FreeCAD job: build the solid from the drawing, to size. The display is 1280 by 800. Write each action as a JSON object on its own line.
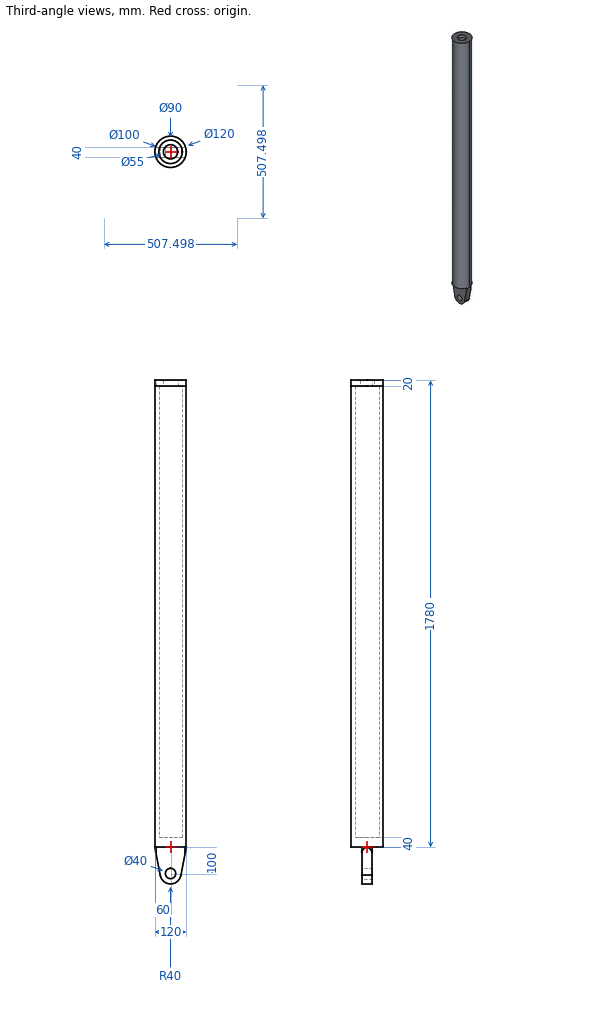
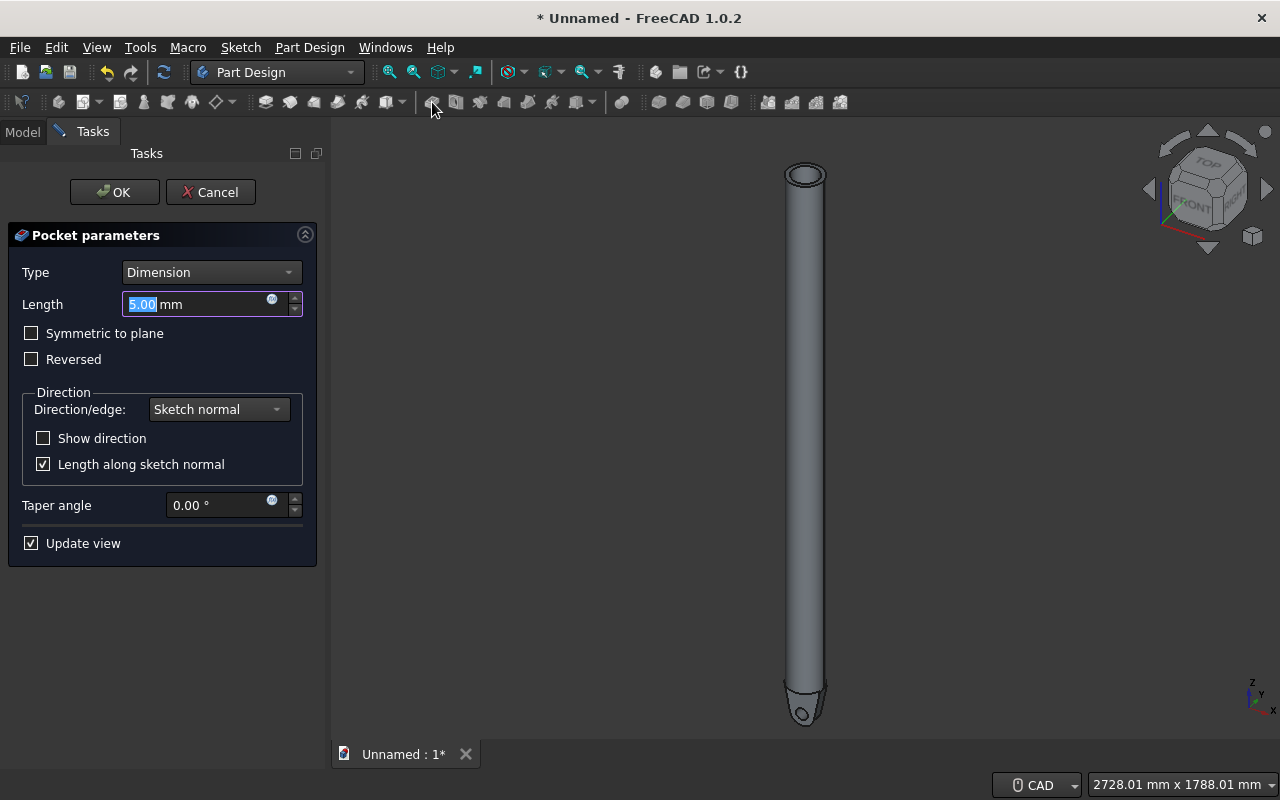
{"action": "left_click", "coordinate": [212, 272]}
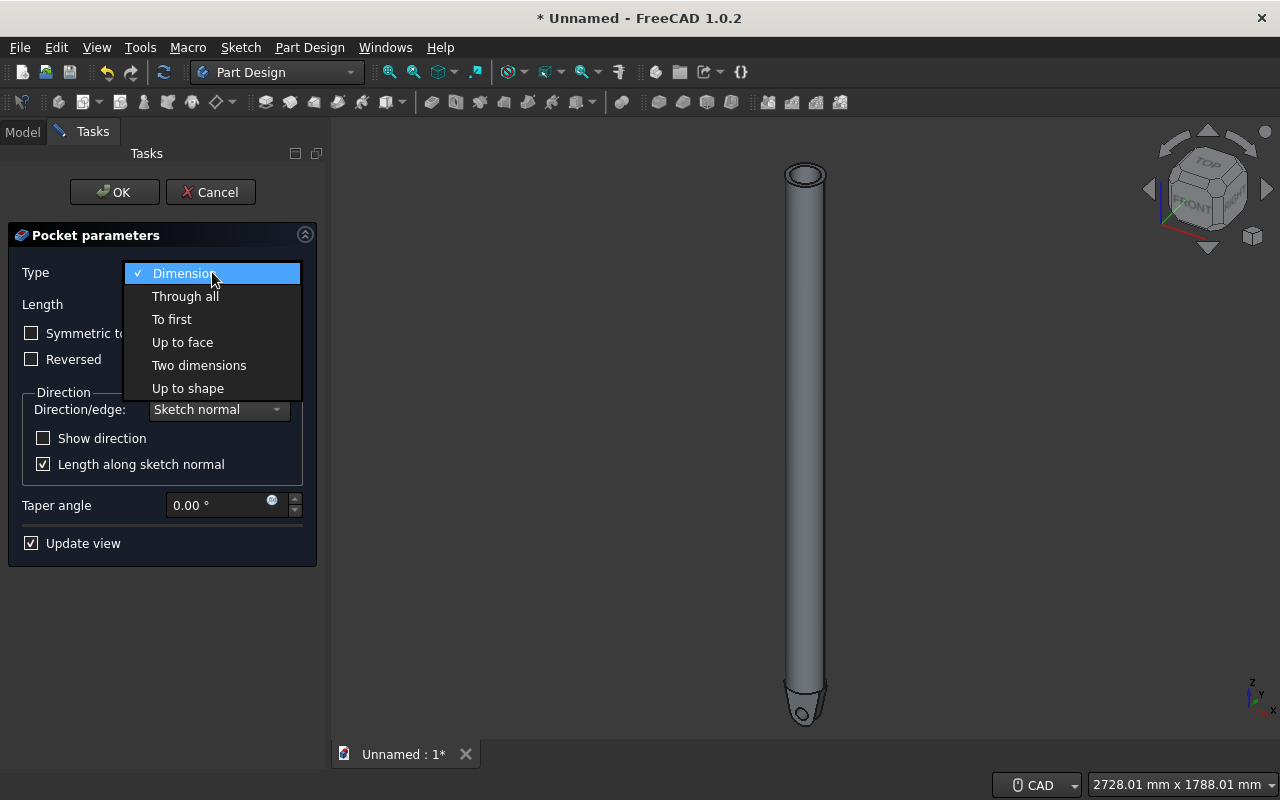
{"action": "left_click", "coordinate": [212, 296]}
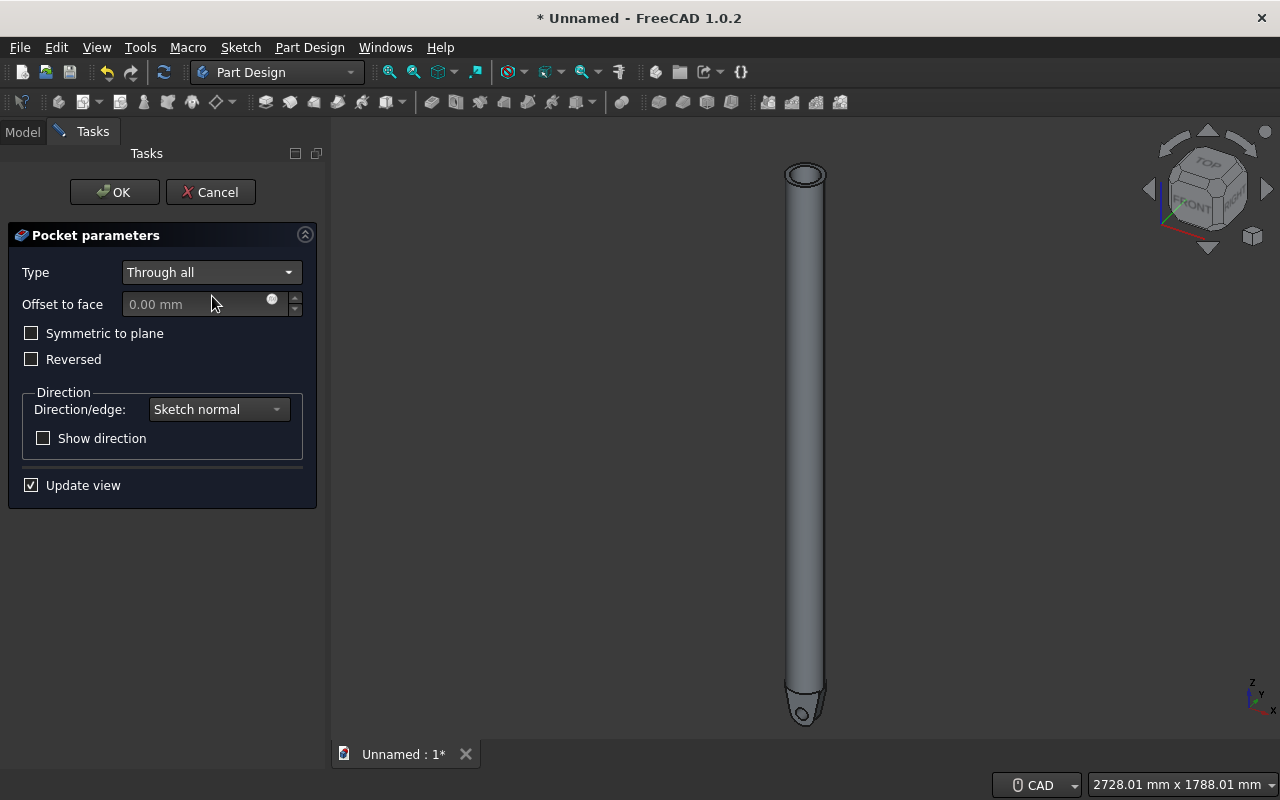
{"action": "left_click", "coordinate": [115, 192]}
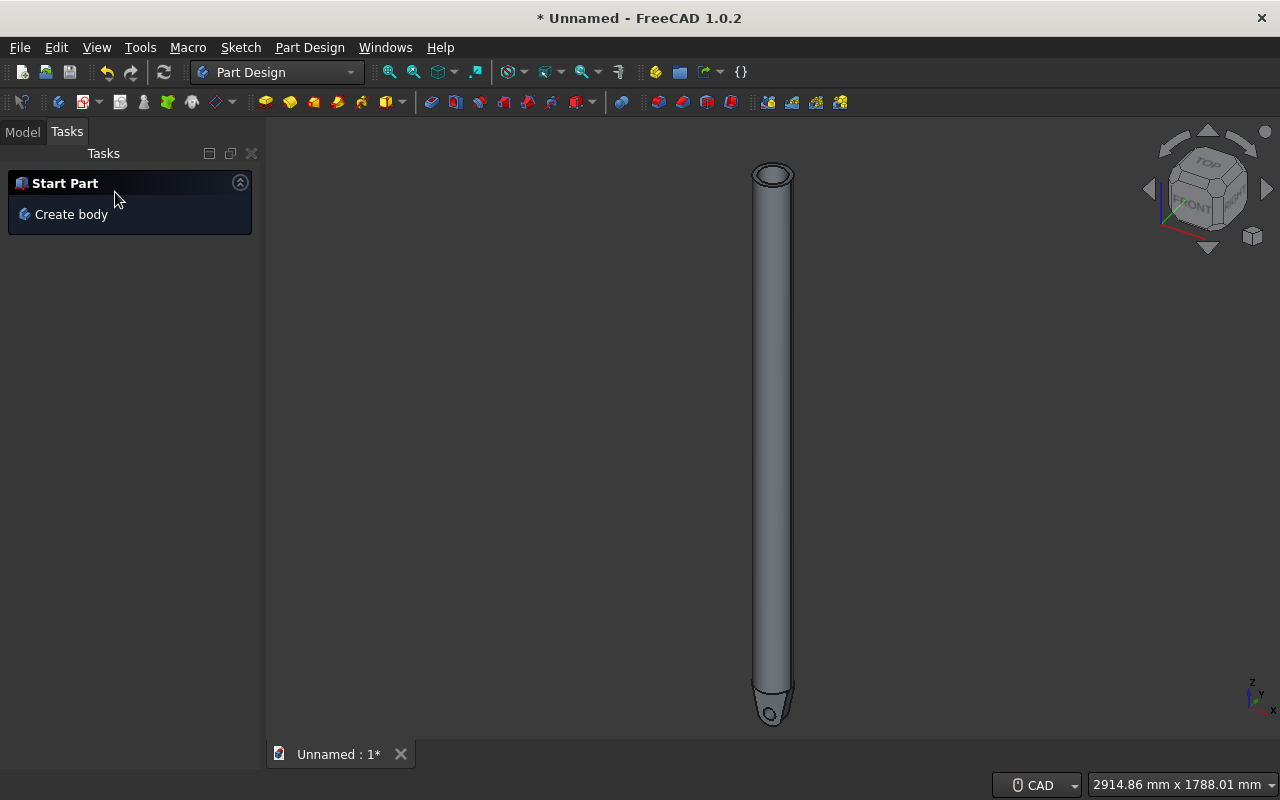
{"action": "left_click", "coordinate": [23, 131]}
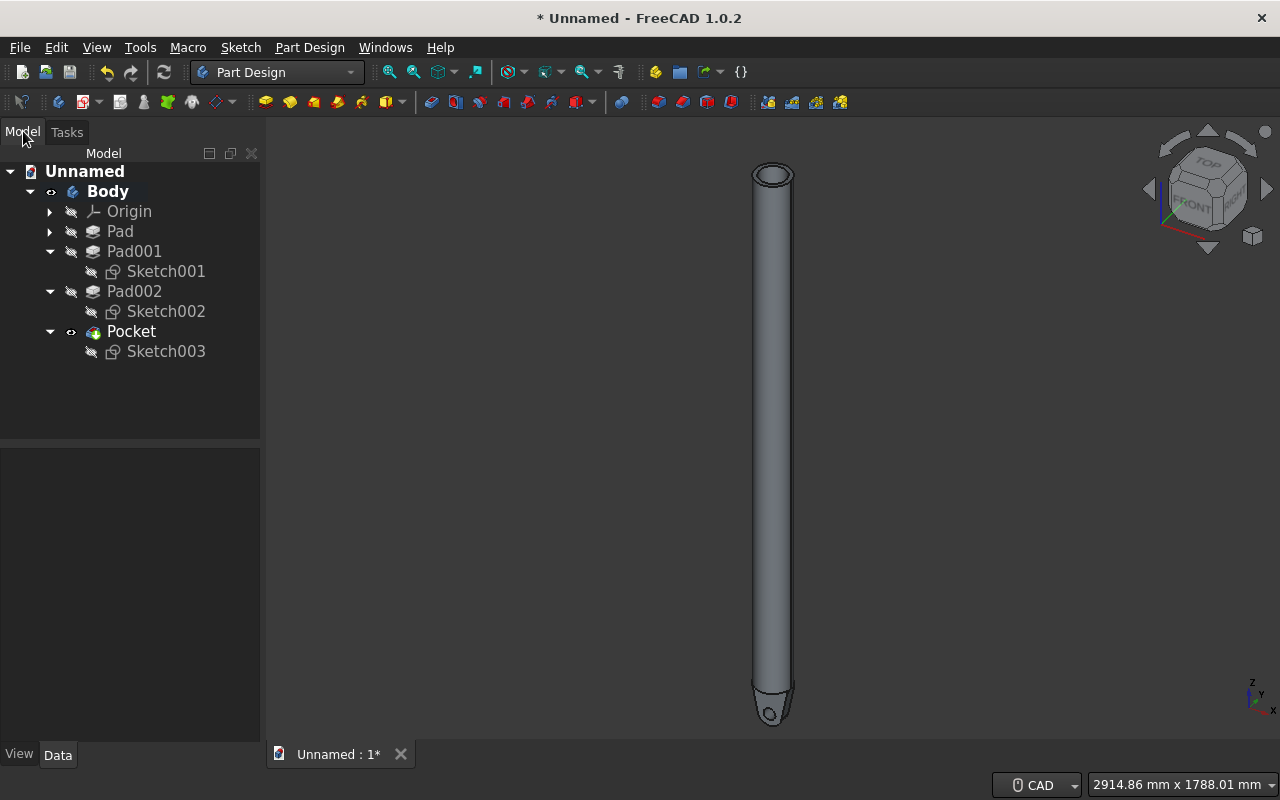
{"action": "left_click", "coordinate": [50, 212]}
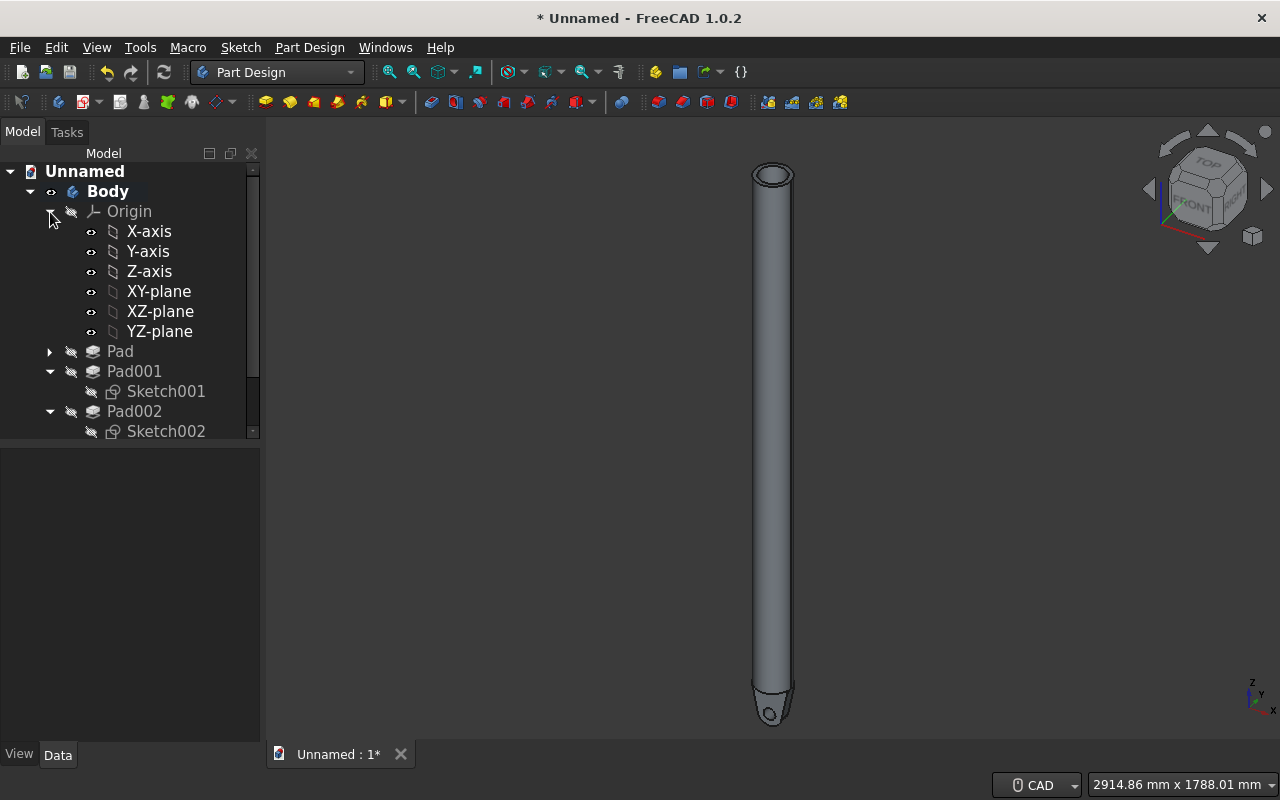
{"action": "left_click", "coordinate": [136, 292]}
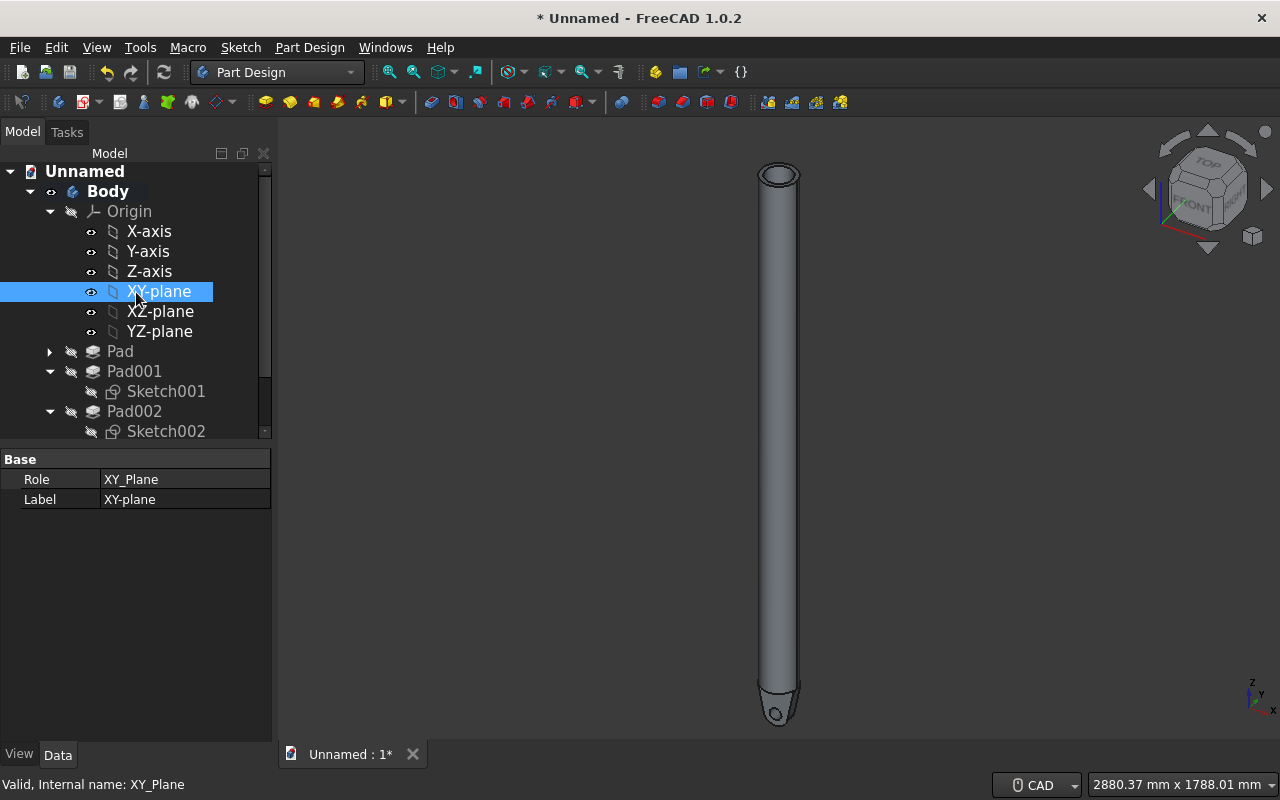
{"action": "left_click", "coordinate": [216, 102]}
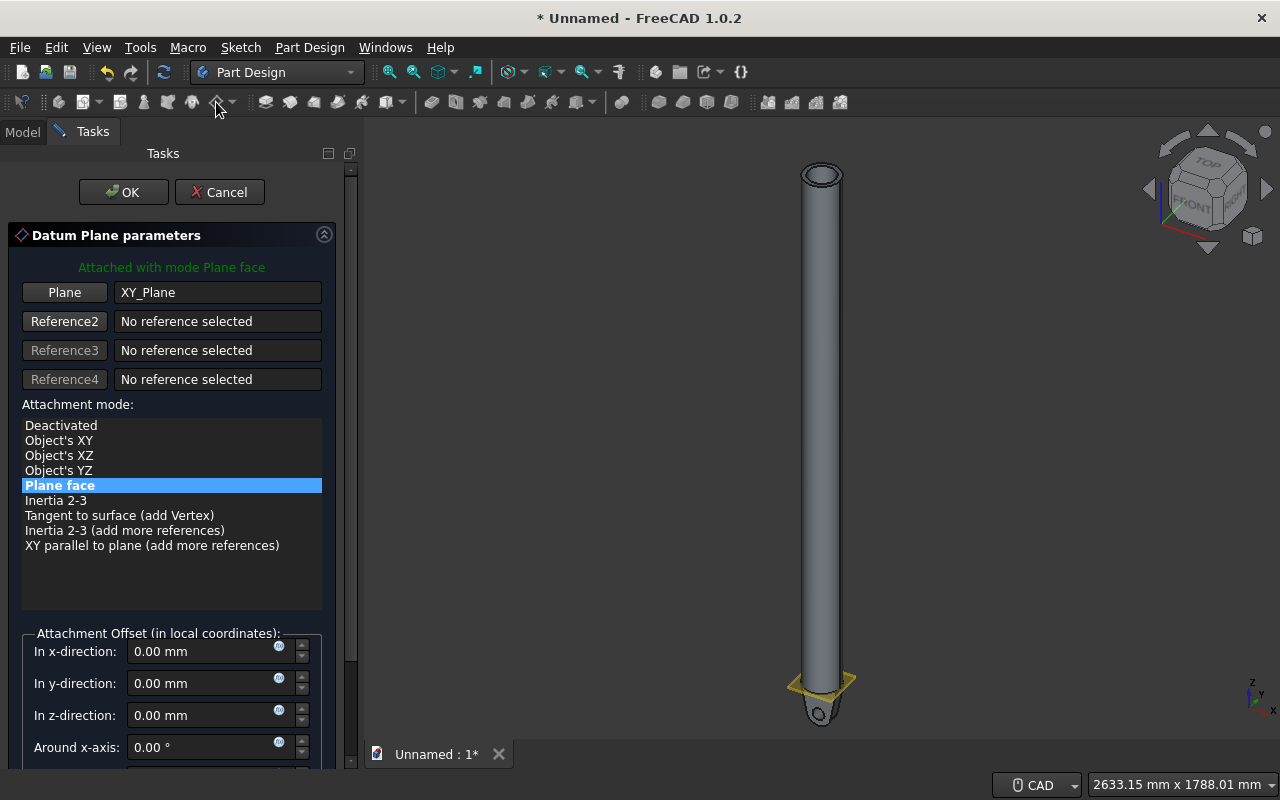
{"action": "triple_click", "coordinate": [210, 715]}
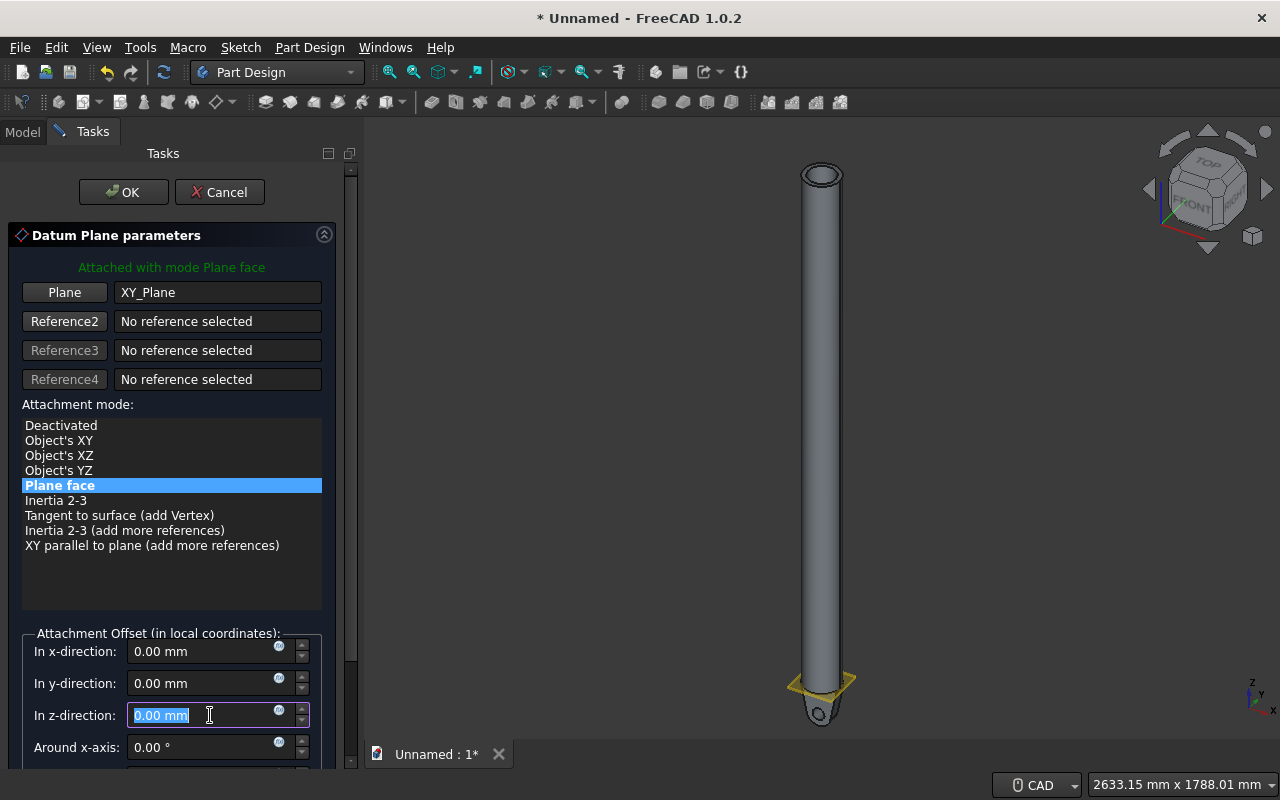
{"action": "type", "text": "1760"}
{"action": "key", "text": "Tab"}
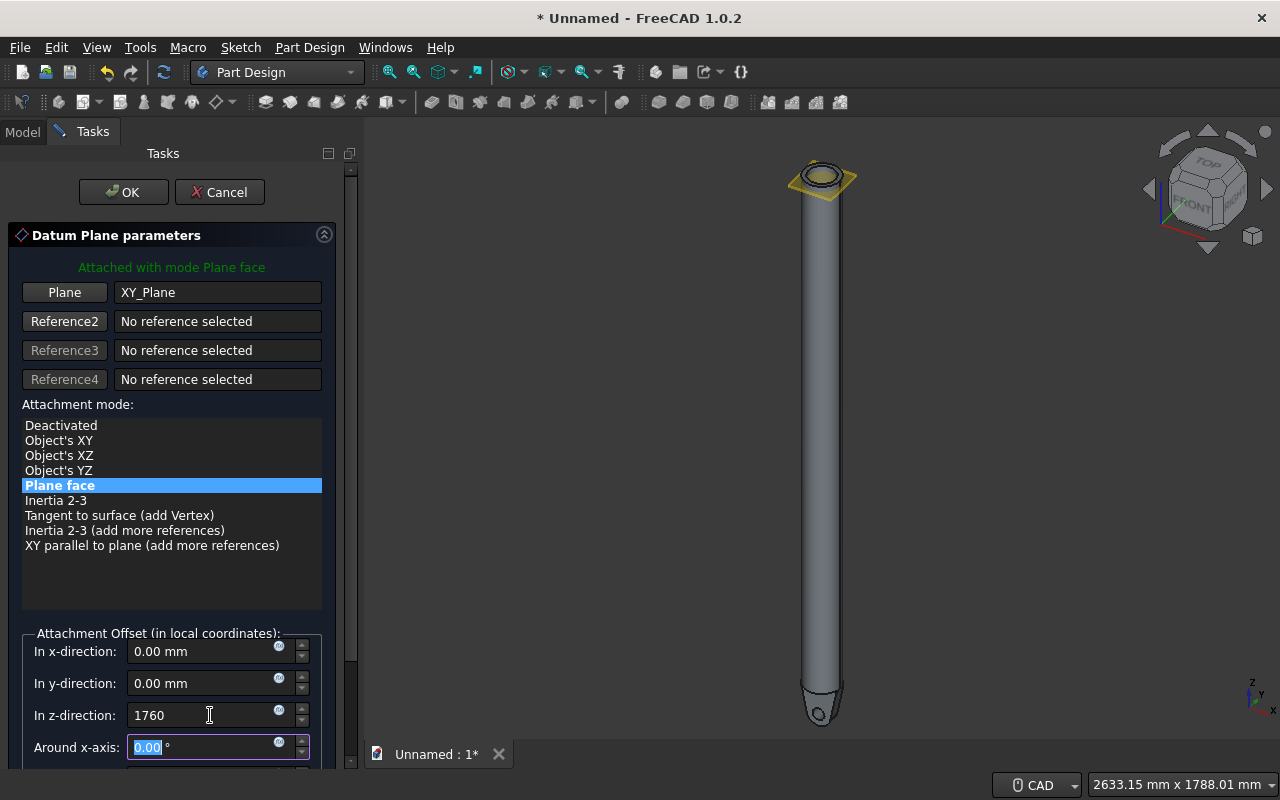
{"action": "left_click", "coordinate": [124, 192]}